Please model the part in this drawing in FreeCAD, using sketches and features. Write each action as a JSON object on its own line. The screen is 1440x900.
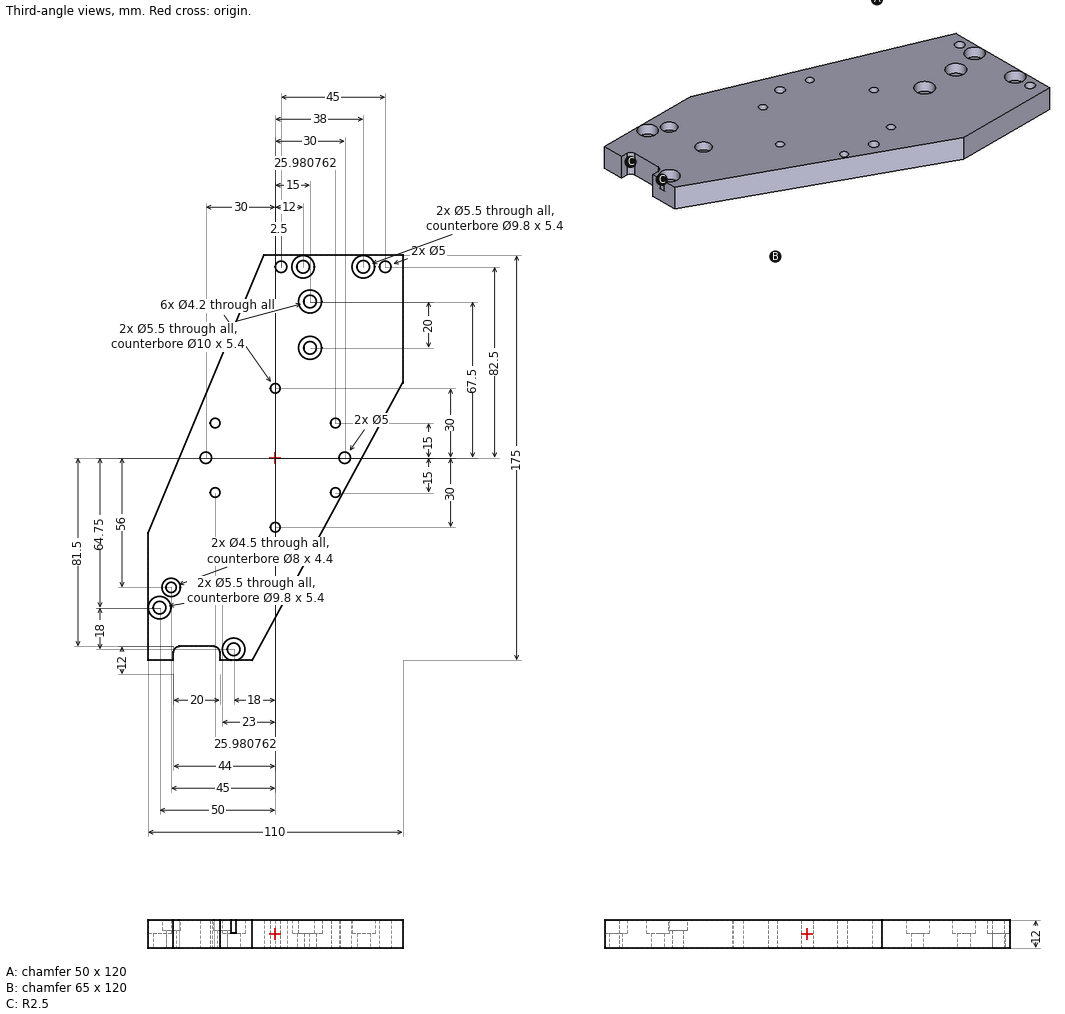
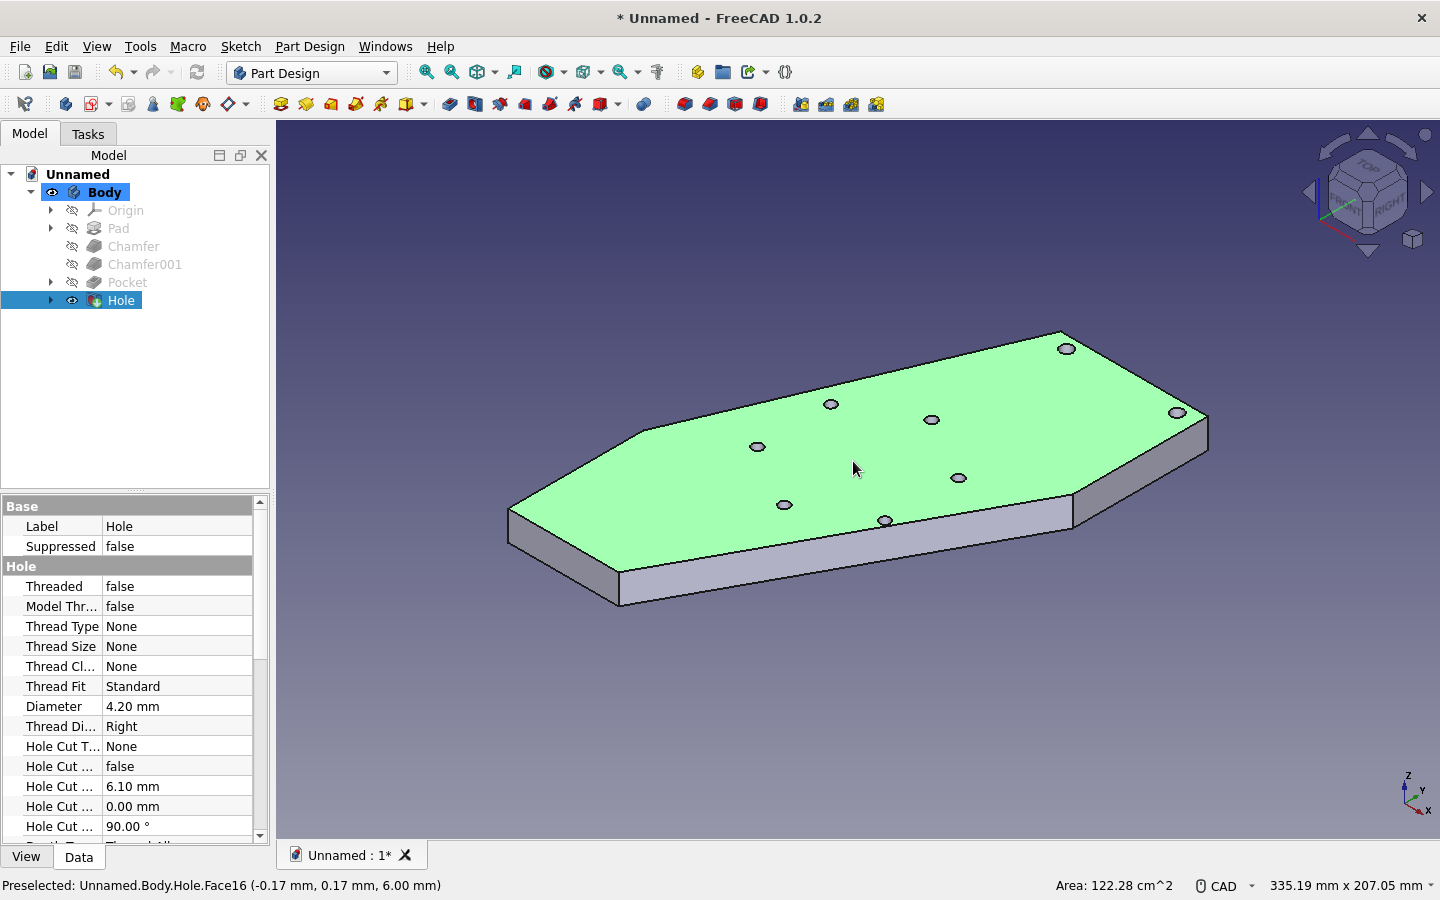
{"action": "left_click", "coordinate": [90, 104]}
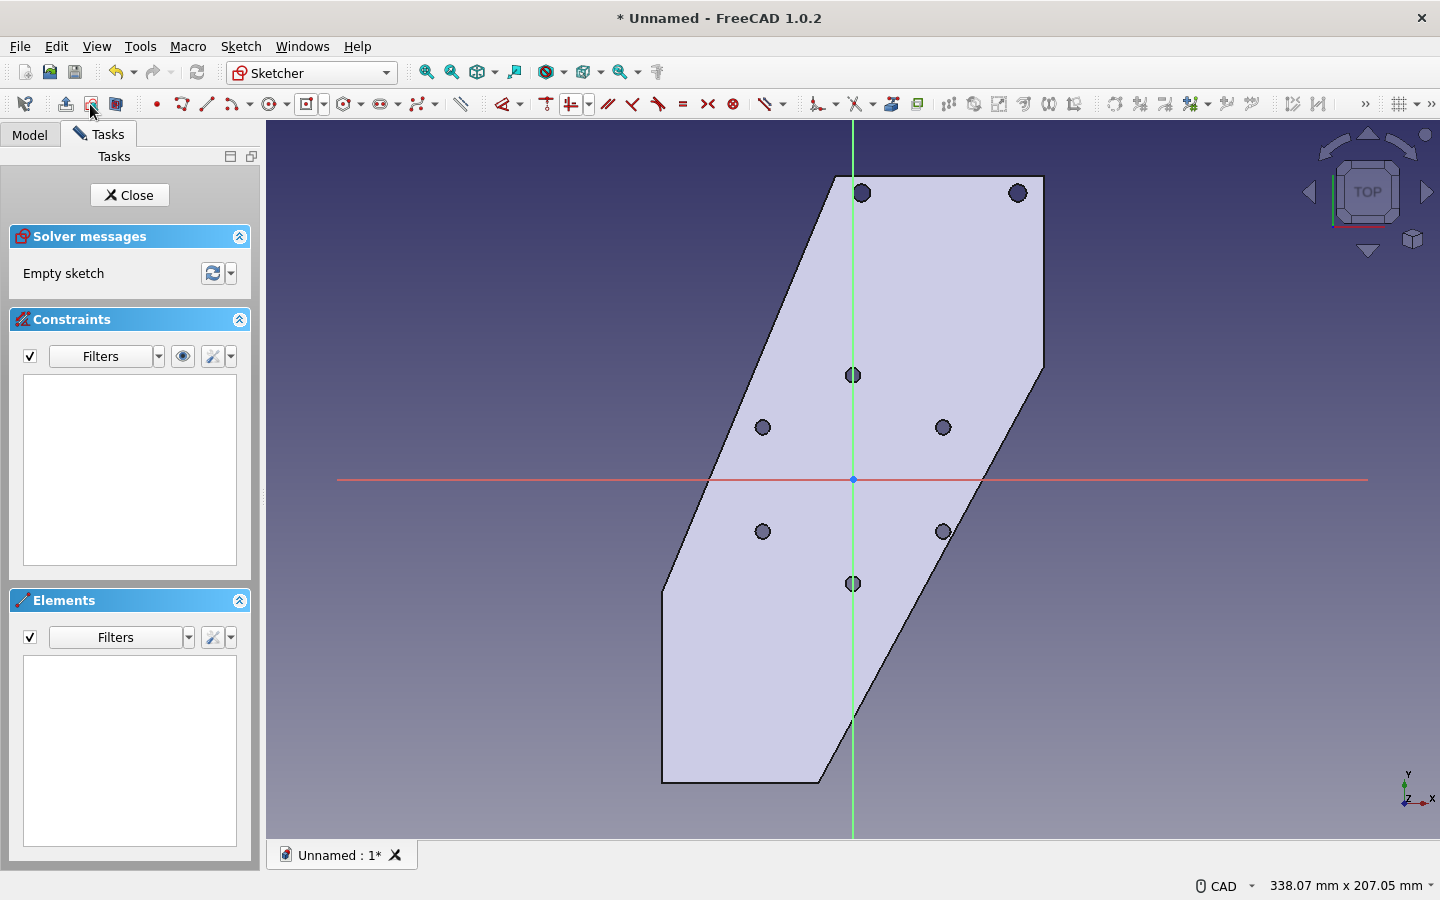
{"action": "scroll", "coordinate": [883, 479], "scroll_direction": "up", "scroll_amount": 6}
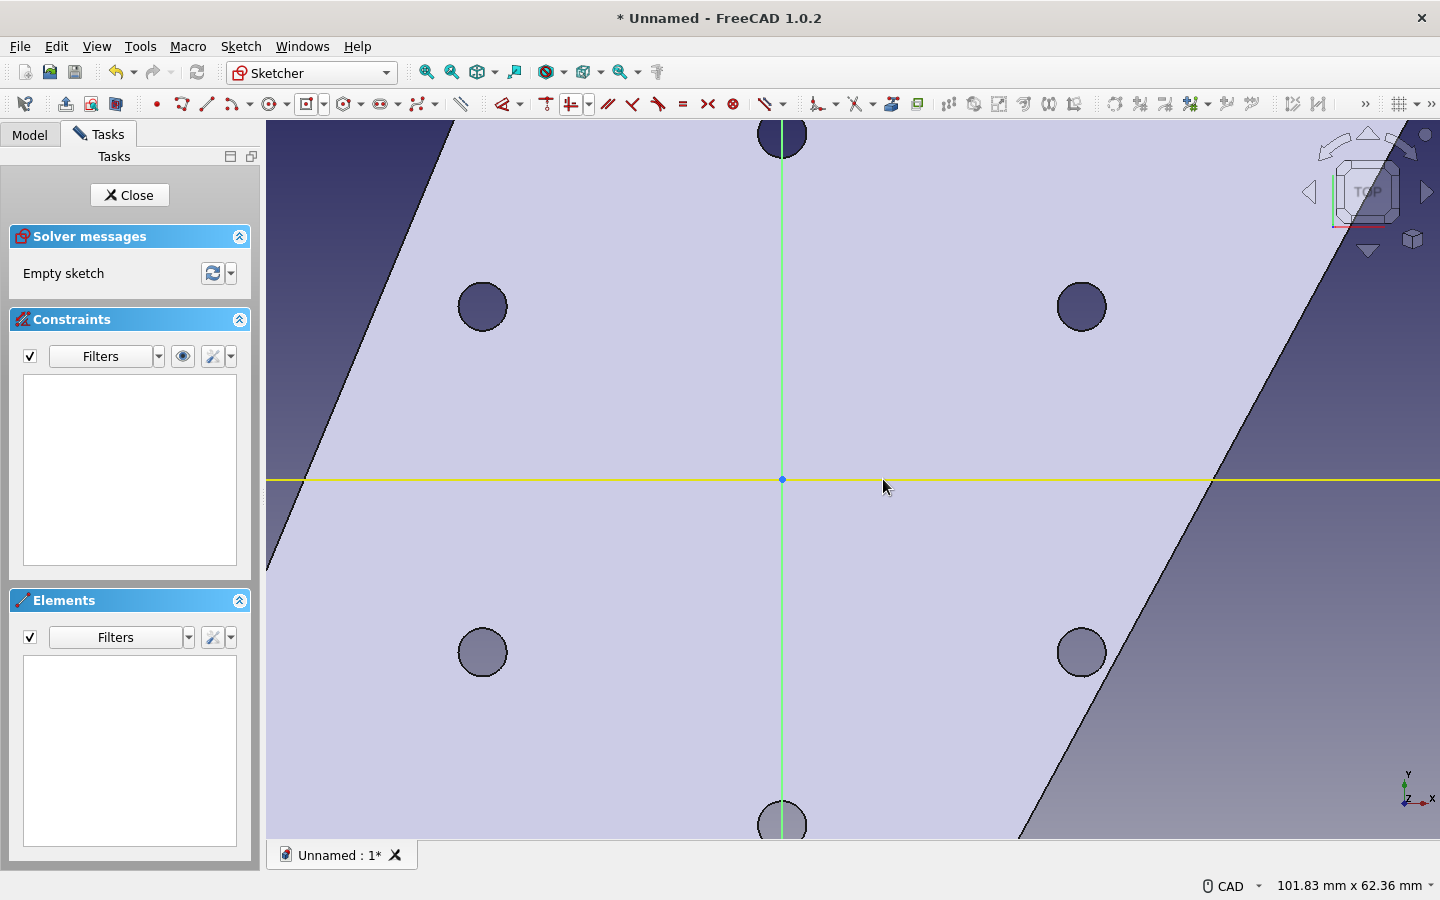
{"action": "key", "text": "g c"}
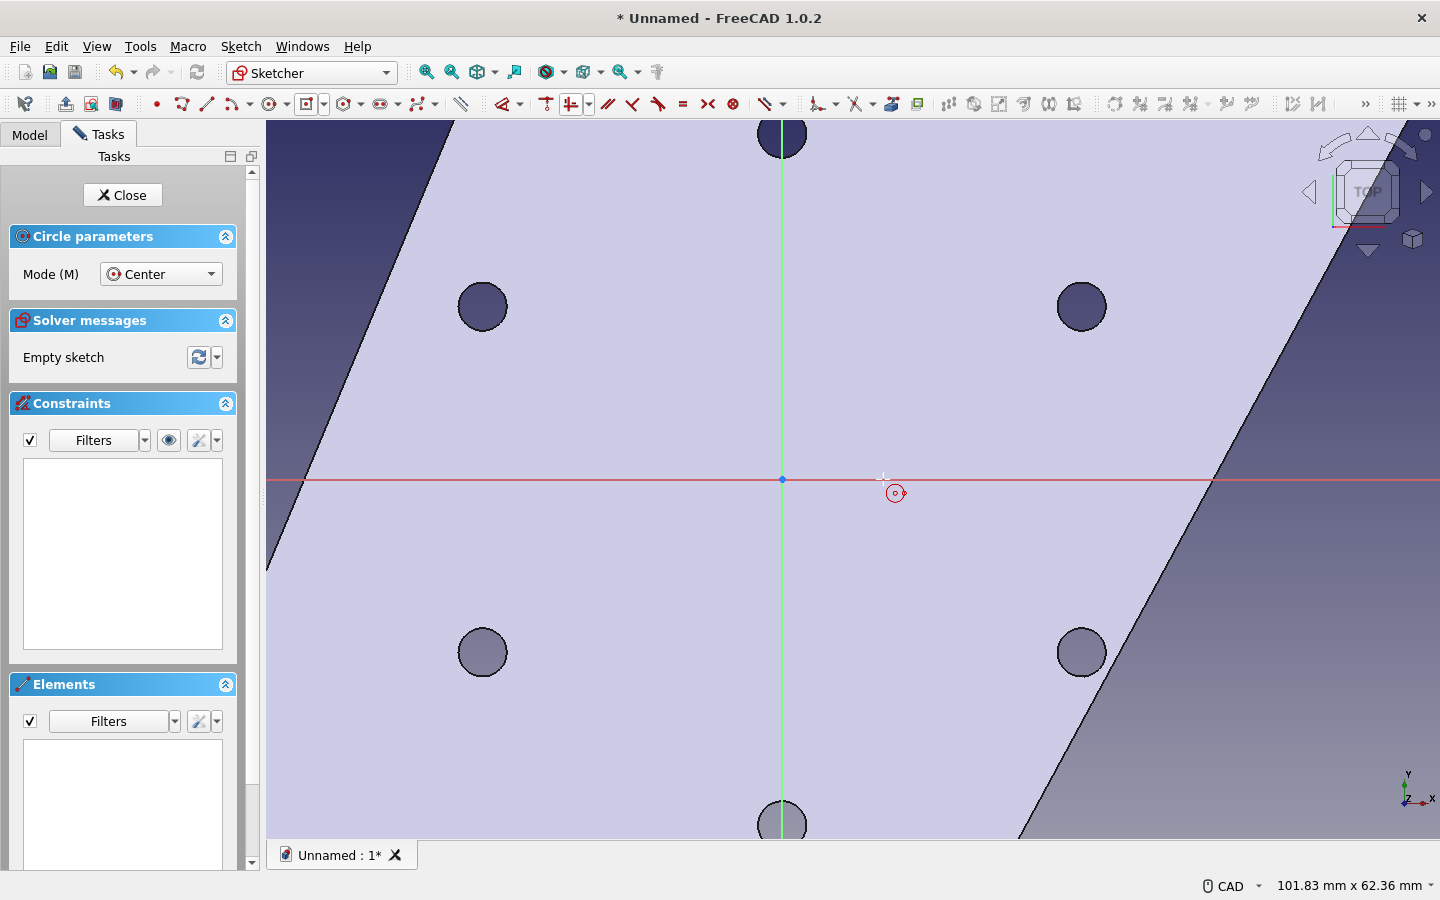
{"action": "left_click", "coordinate": [1128, 479]}
{"action": "left_click", "coordinate": [1148, 459]}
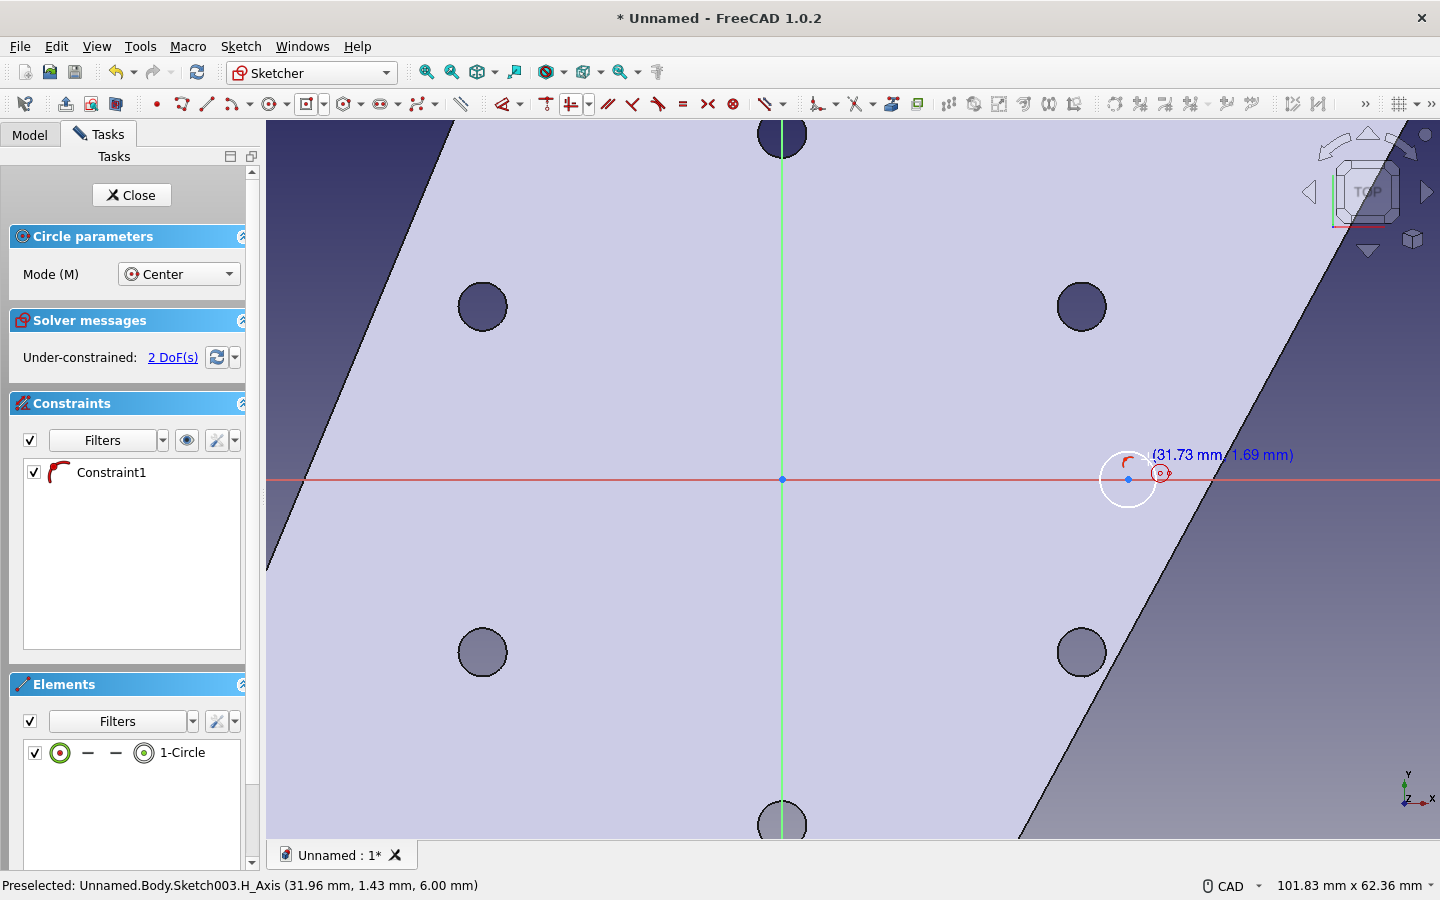
{"action": "left_click", "coordinate": [436, 479]}
{"action": "left_click", "coordinate": [457, 459]}
{"action": "key", "text": "Escape"}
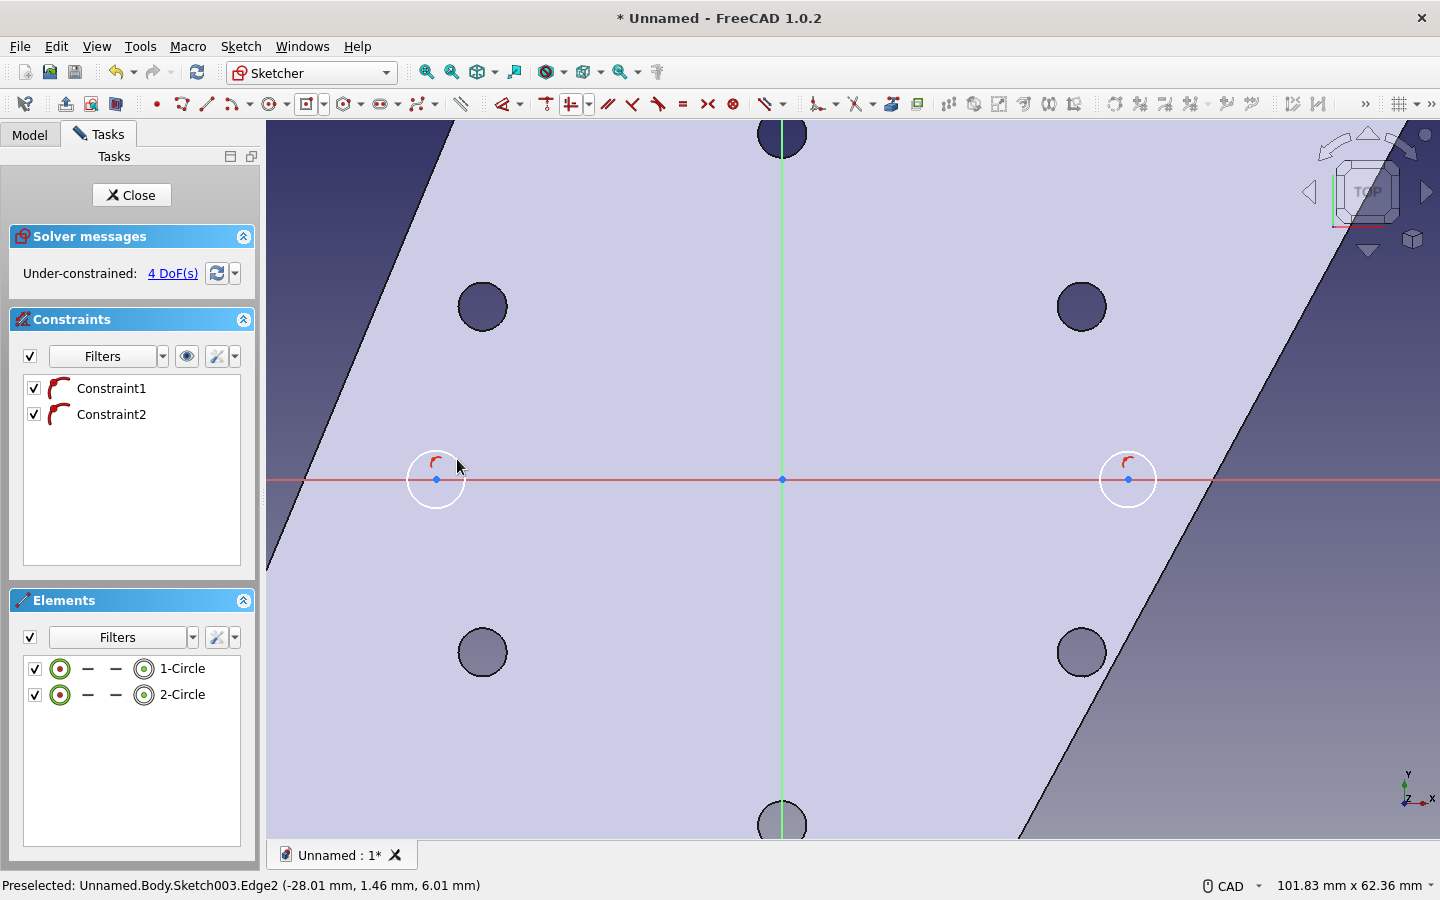
{"action": "left_click", "coordinate": [1148, 460]}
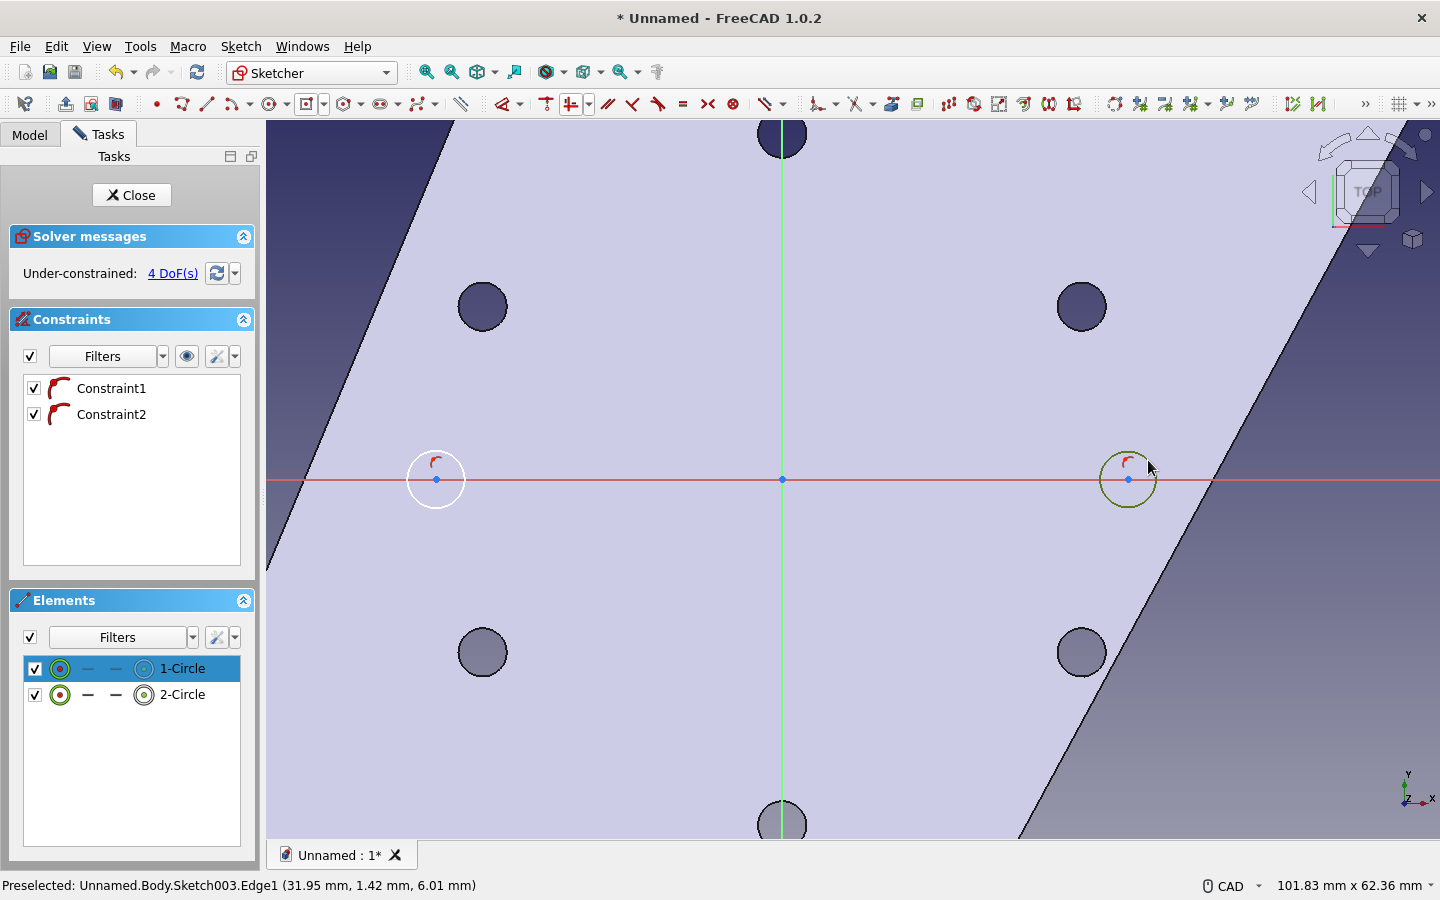
{"action": "left_click", "coordinate": [456, 459]}